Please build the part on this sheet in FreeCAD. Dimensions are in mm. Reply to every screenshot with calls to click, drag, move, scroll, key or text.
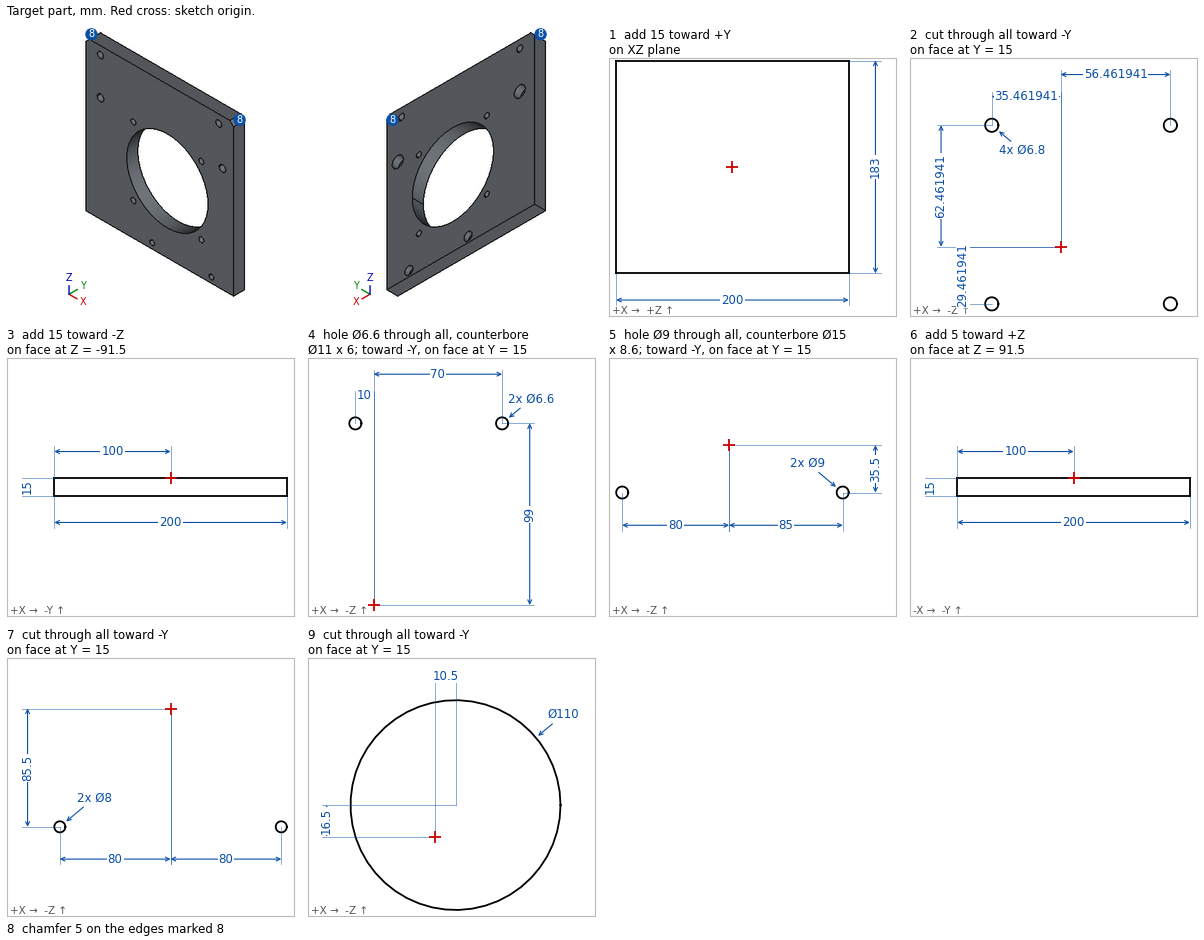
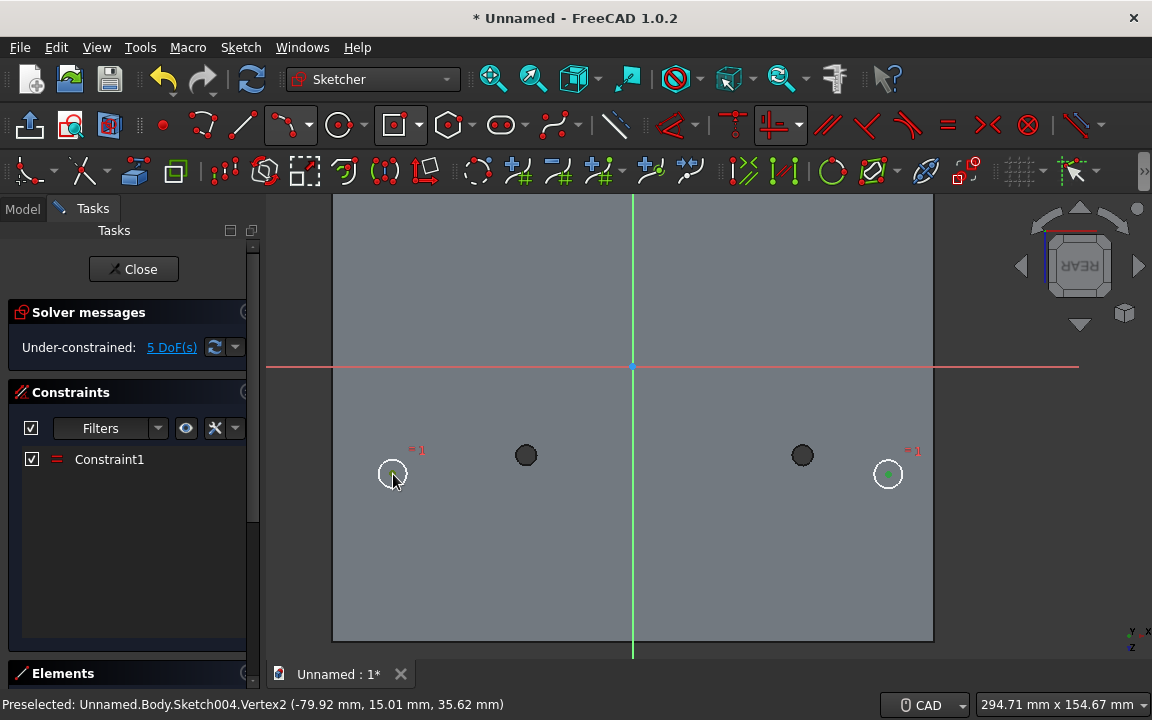
key(h)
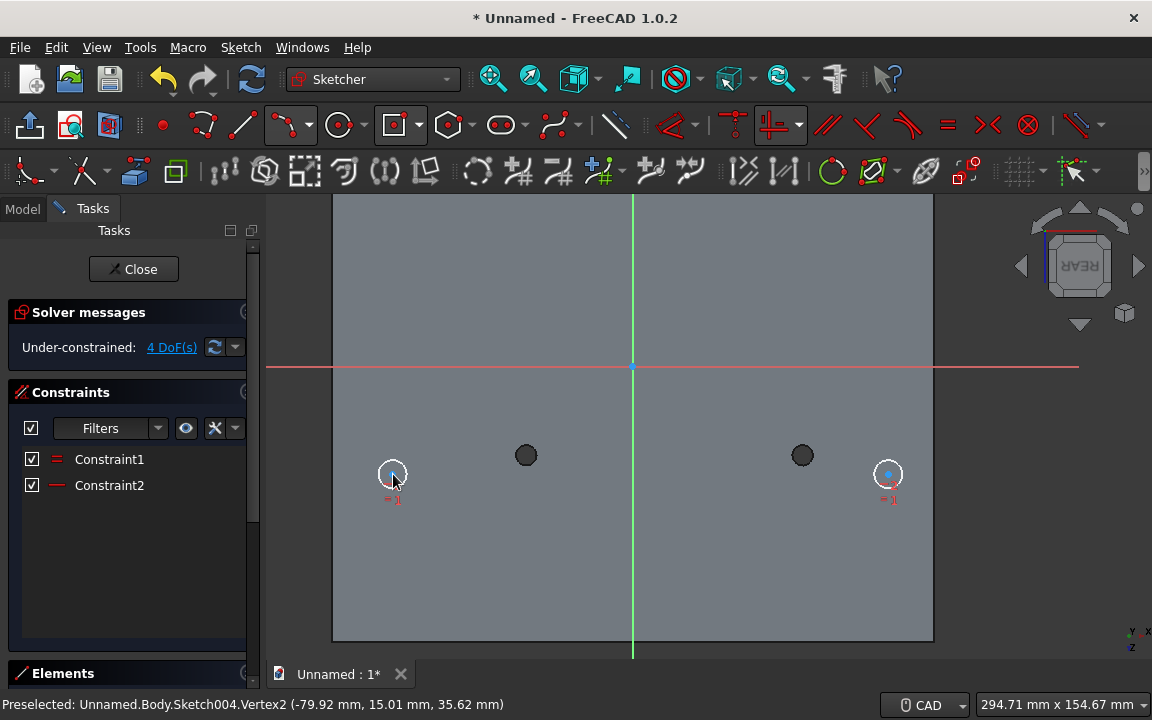
click(670, 126)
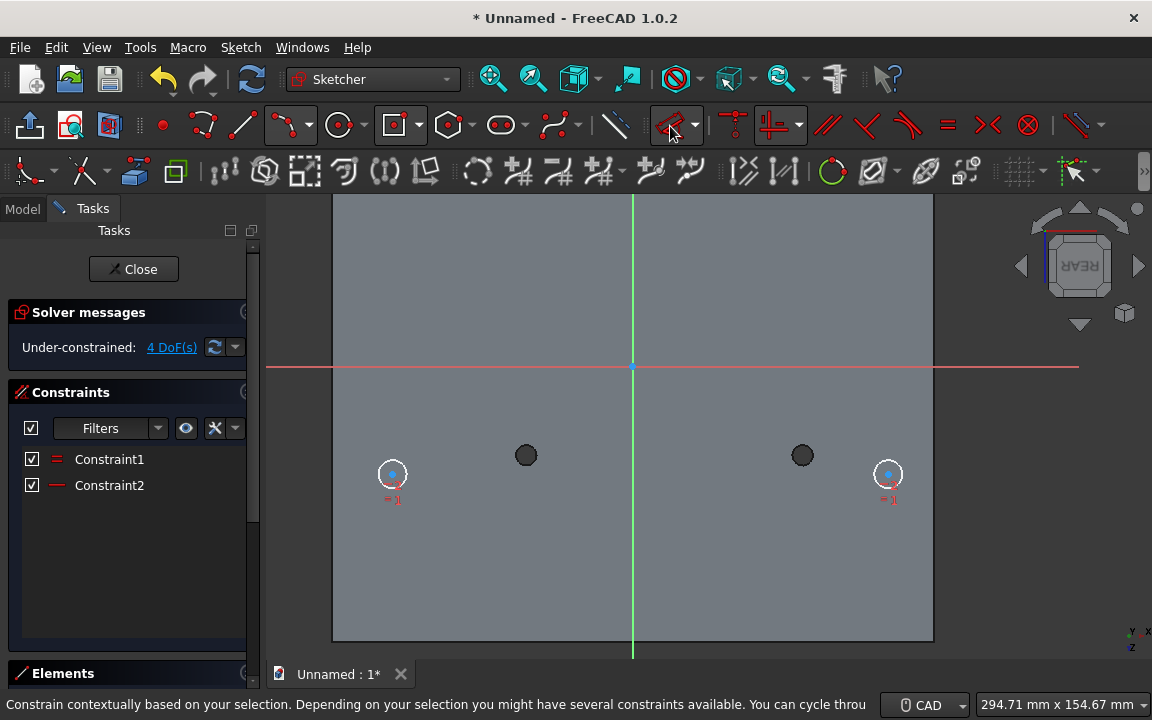
scroll(898, 464, up, 2)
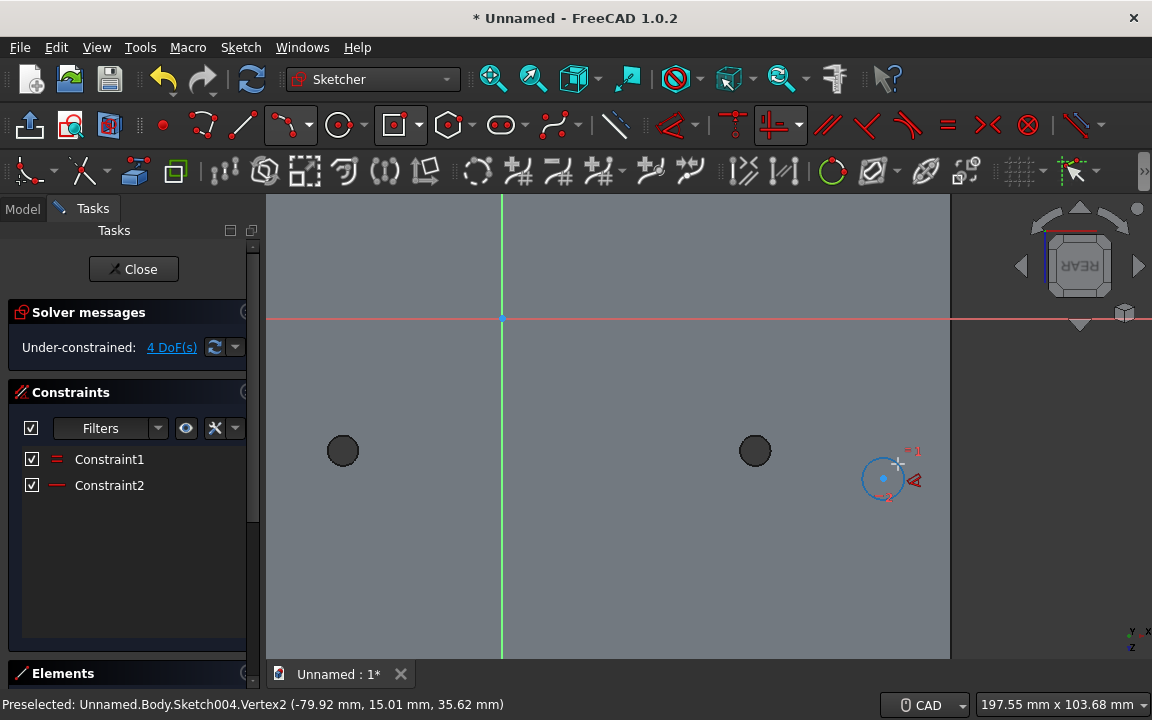
click(898, 464)
click(921, 441)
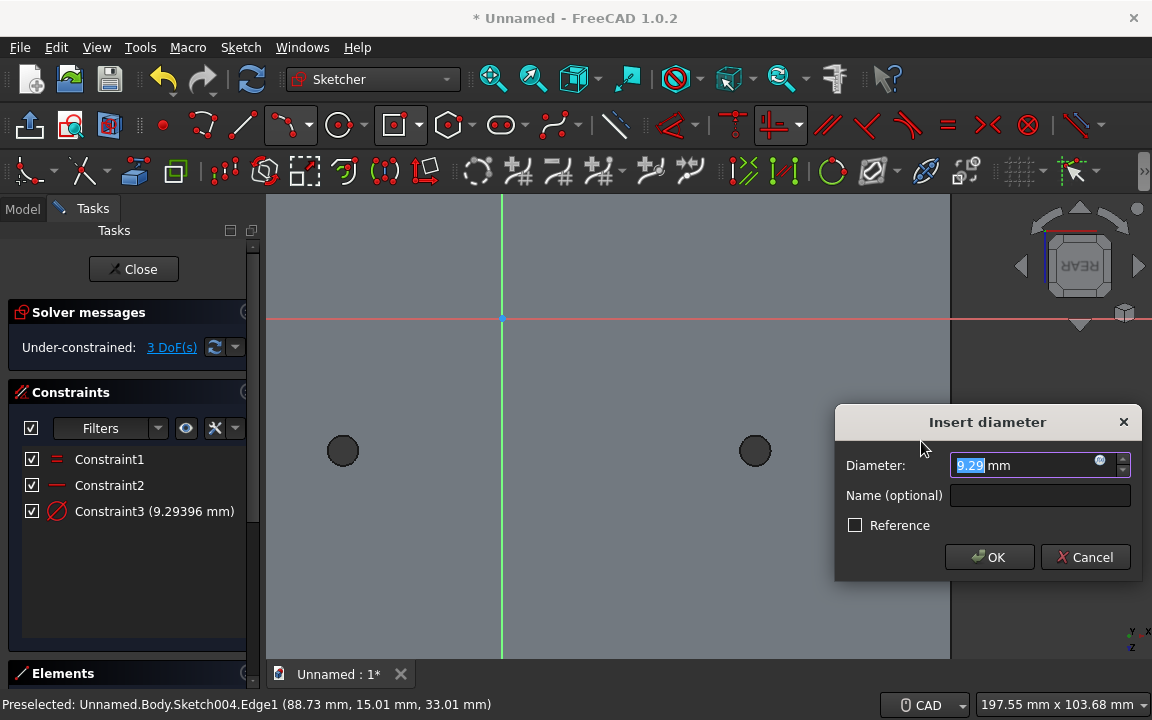
text(9)
key(Return)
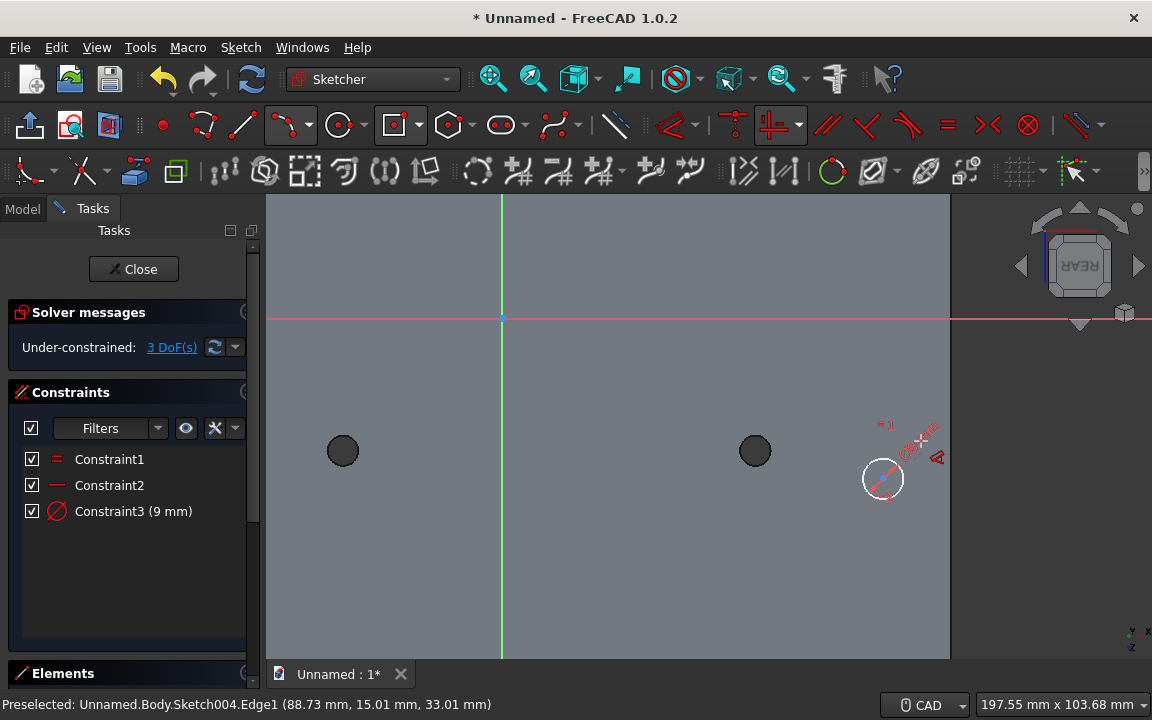
click(883, 479)
click(693, 285)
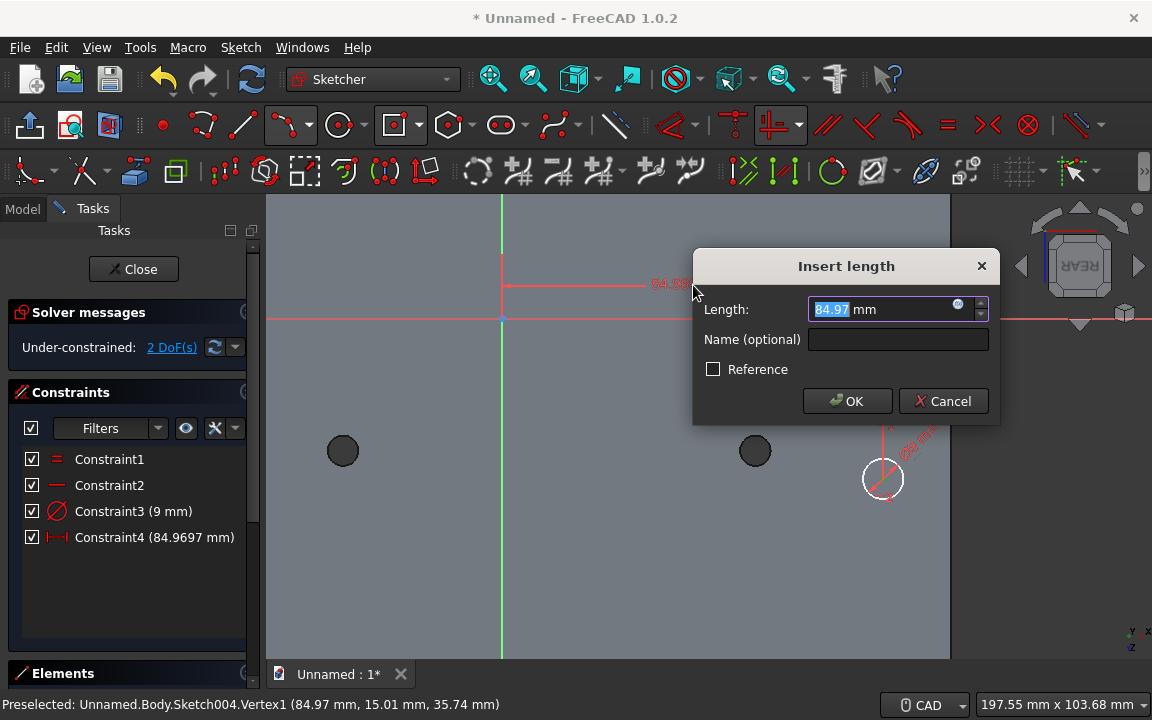
text(85)
key(Return)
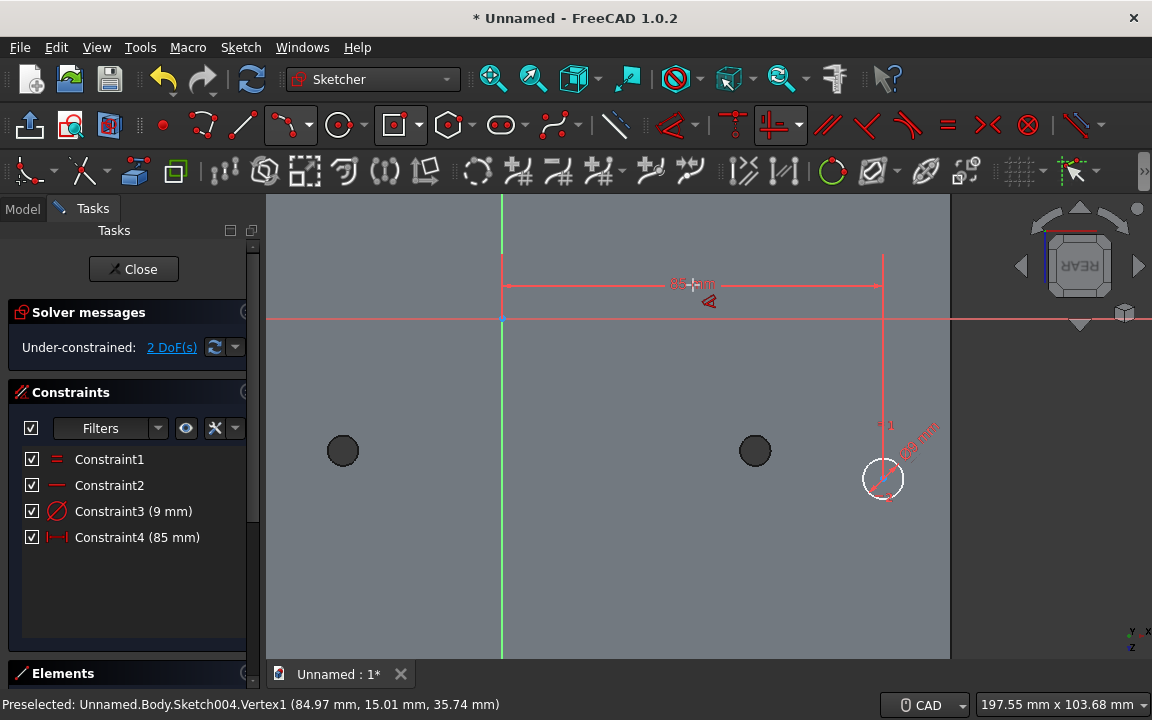
scroll(899, 463, down, 2)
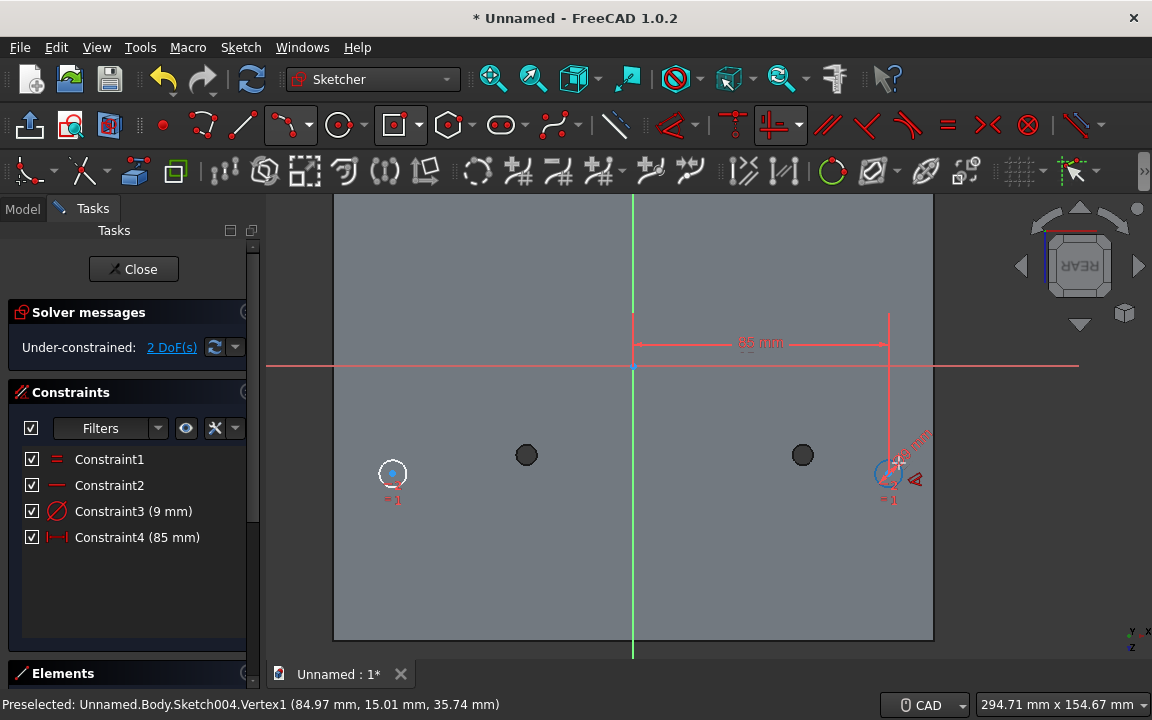
click(393, 474)
click(513, 332)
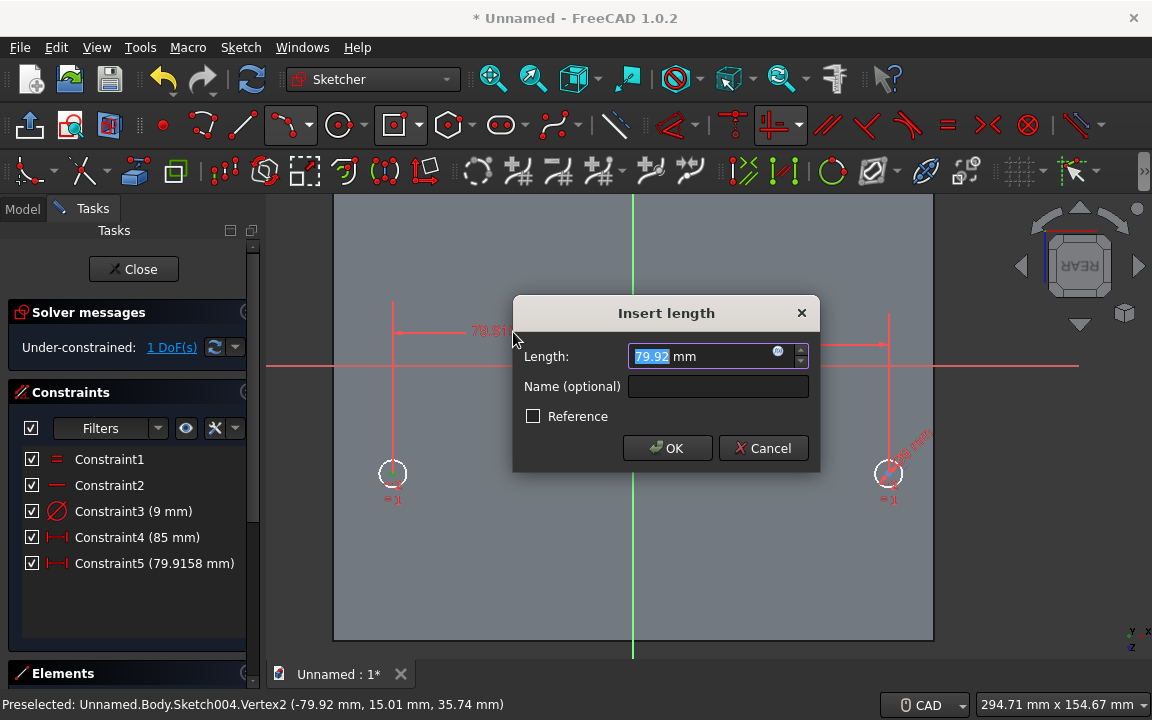
text(80)
key(Return)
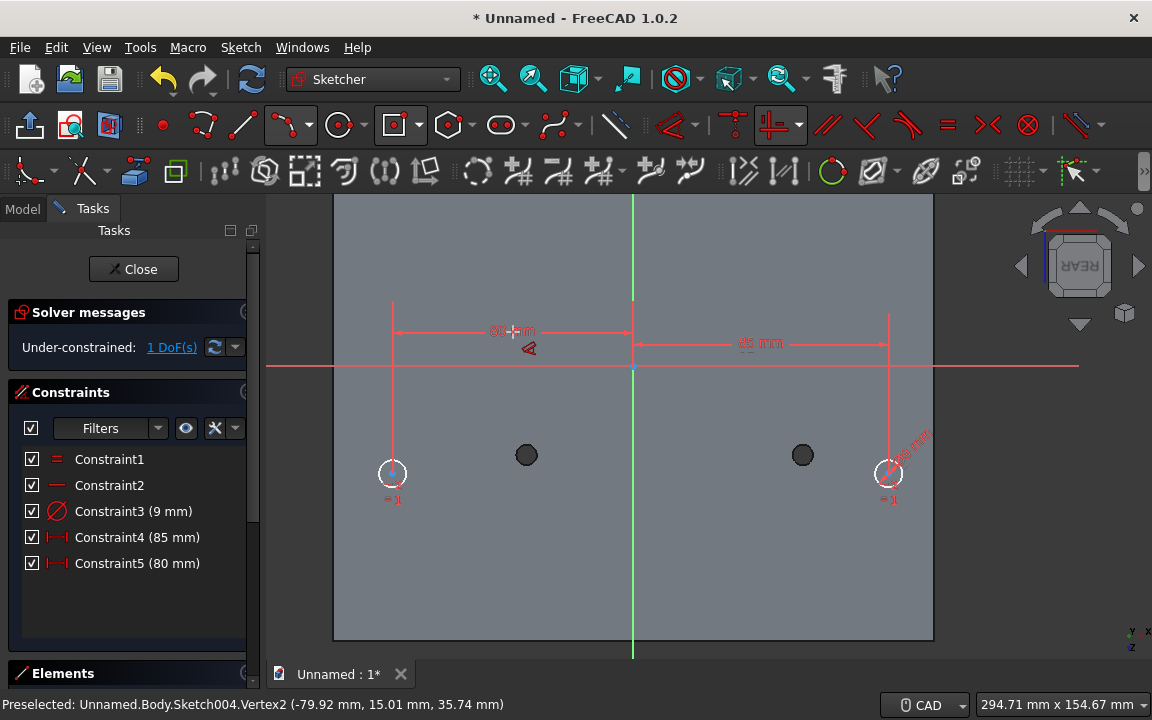
click(889, 474)
click(923, 420)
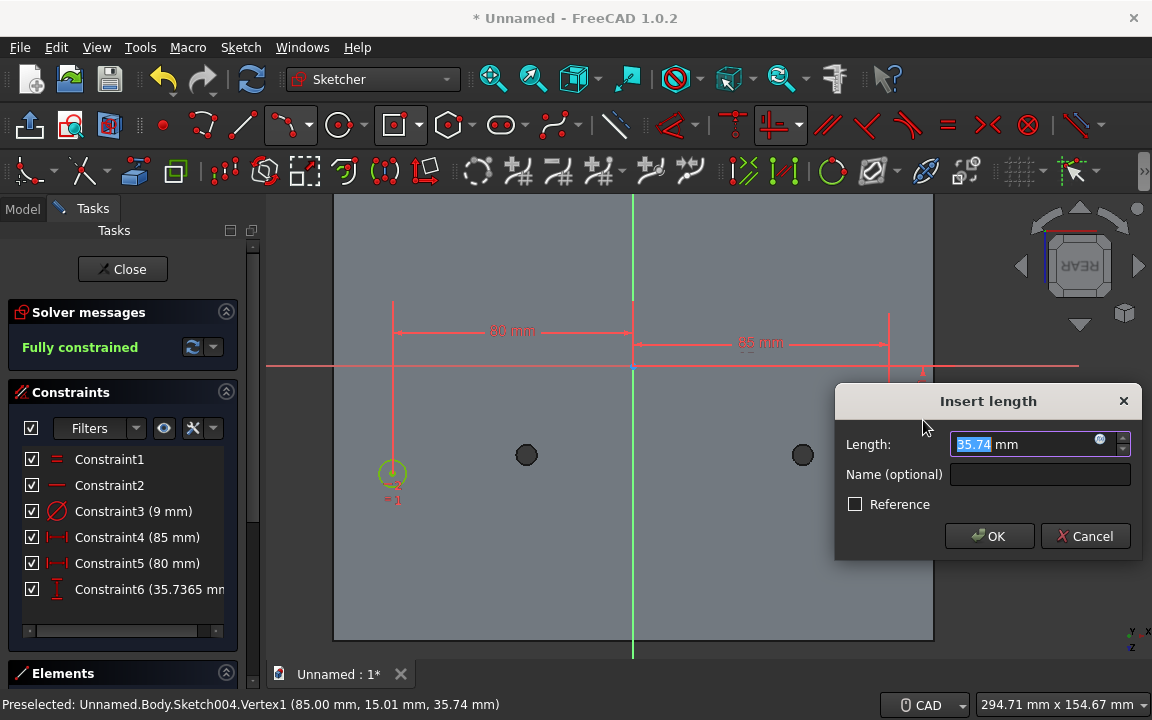
text(35.5)
key(Return)
key(Escape)